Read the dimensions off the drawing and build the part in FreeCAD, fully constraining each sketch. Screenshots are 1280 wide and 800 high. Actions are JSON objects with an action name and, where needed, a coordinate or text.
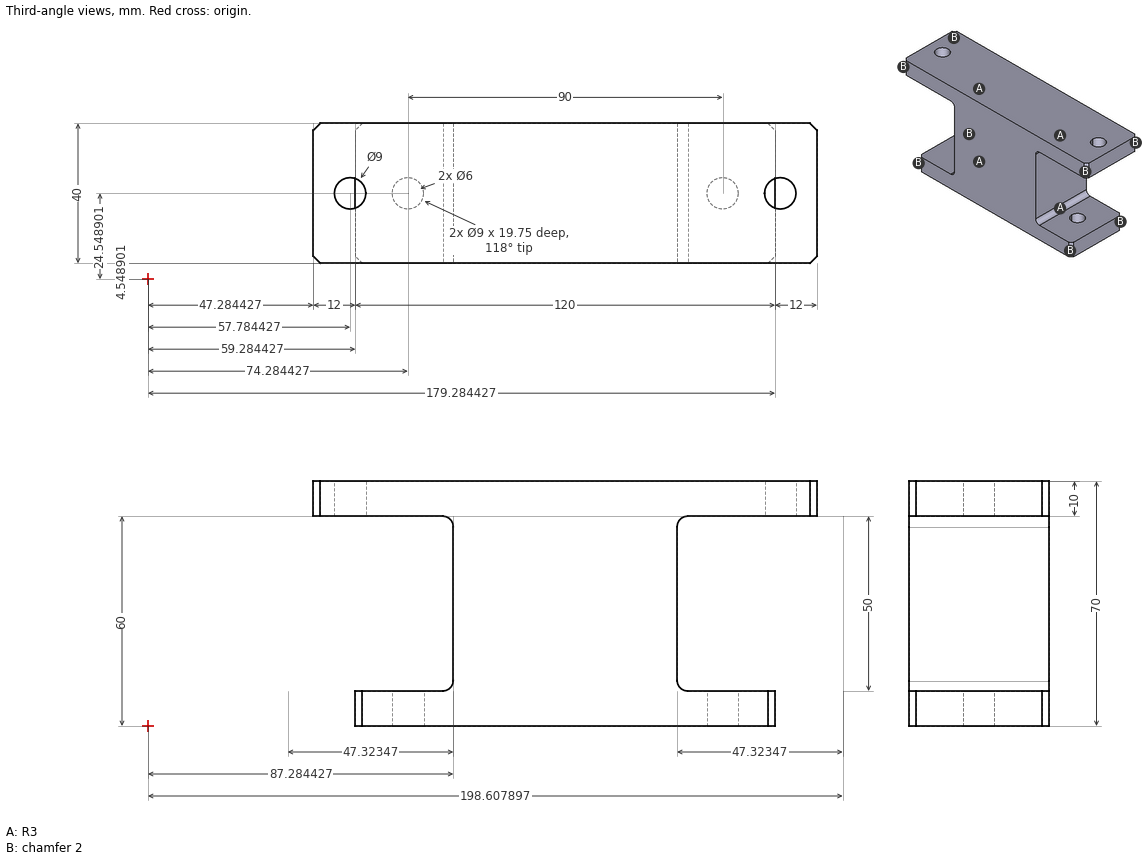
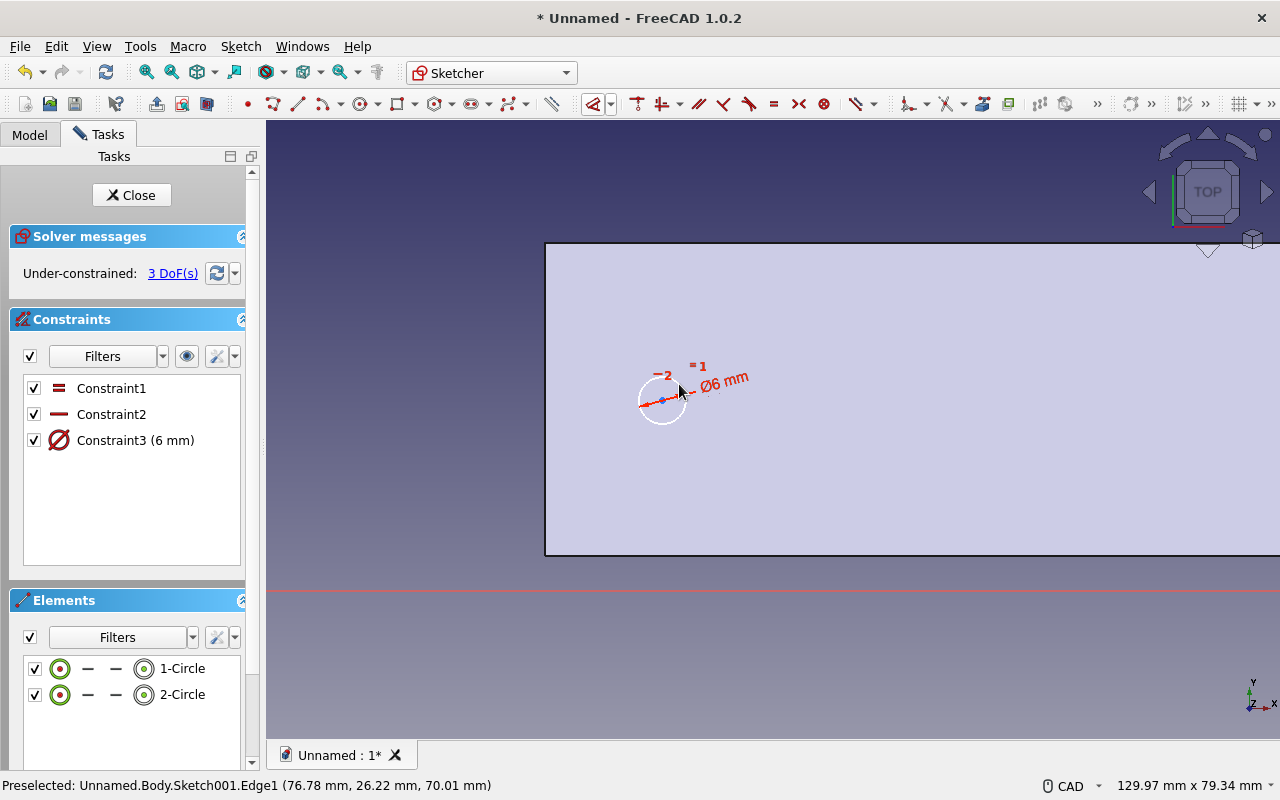
{"action": "left_click", "coordinate": [662, 401]}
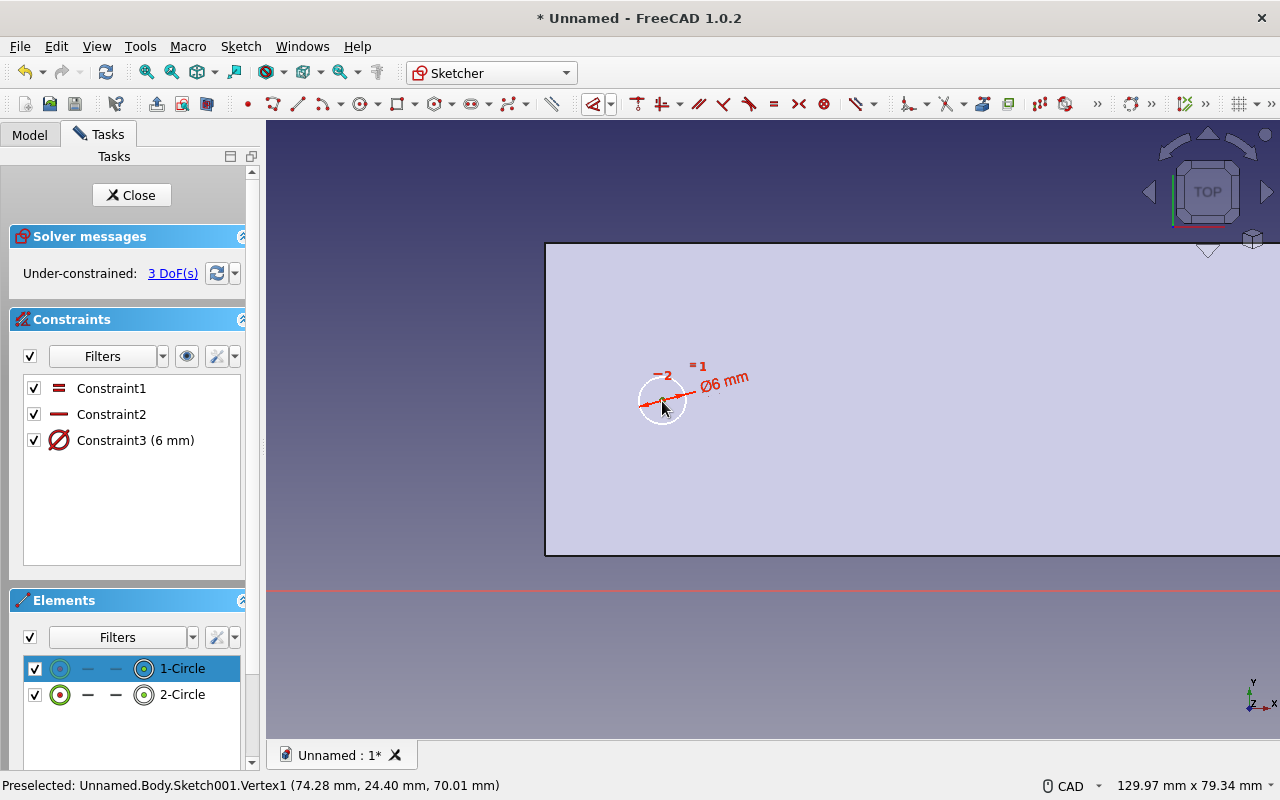
{"action": "scroll", "coordinate": [679, 385], "scroll_direction": "down", "scroll_amount": 4}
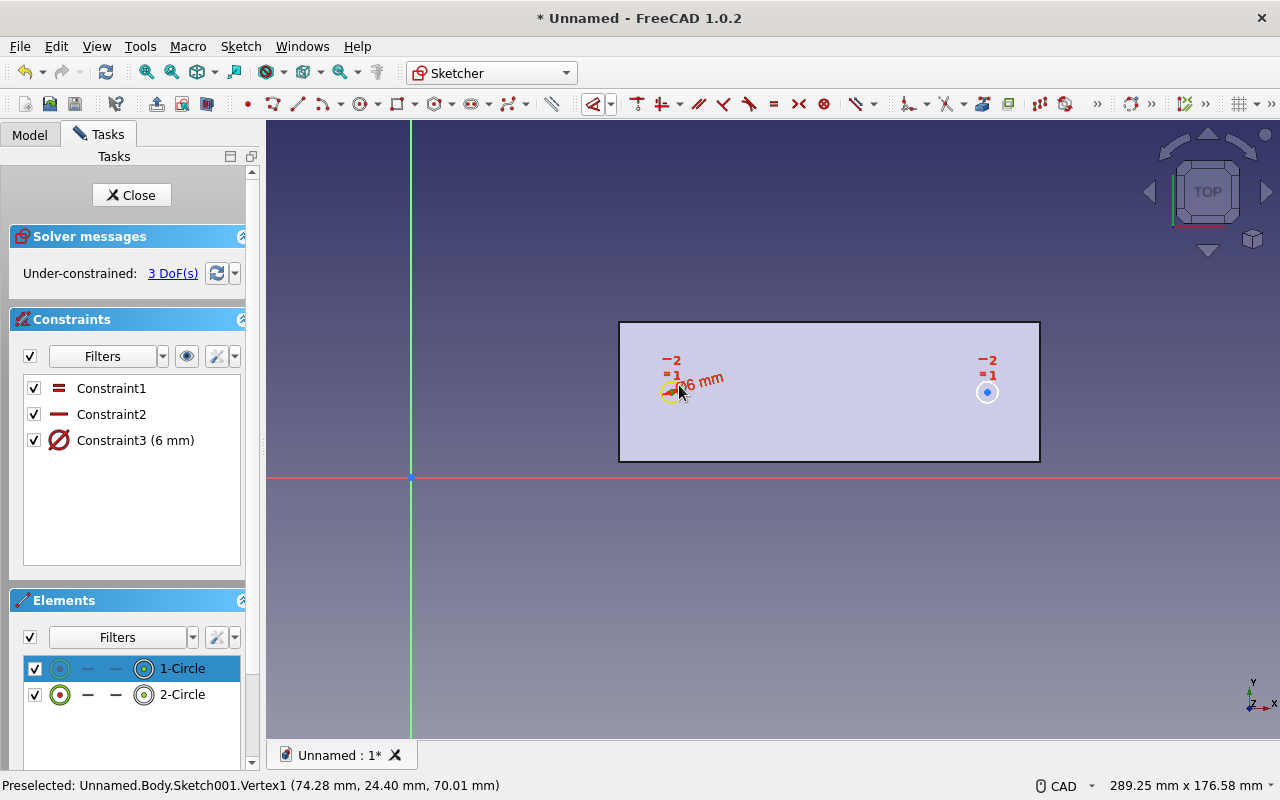
{"action": "left_click", "coordinate": [987, 392]}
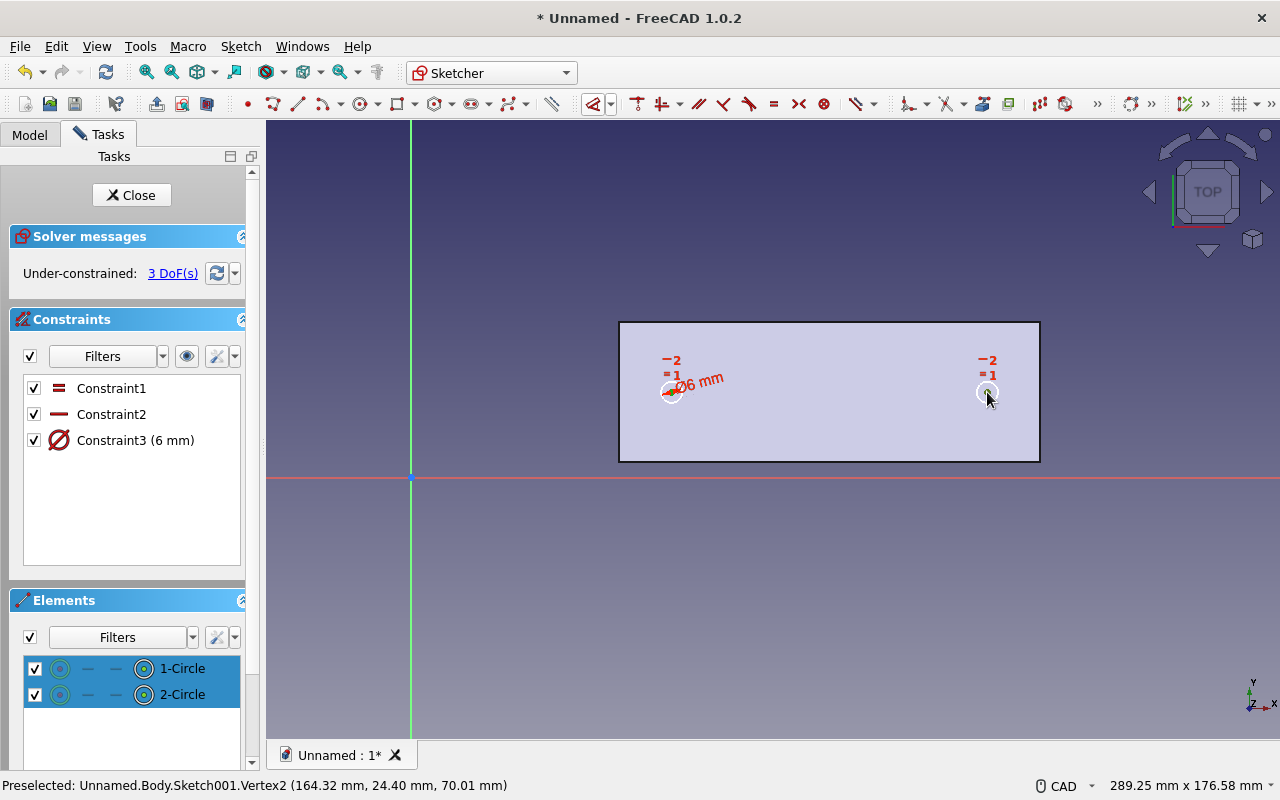
{"action": "key", "text": "l"}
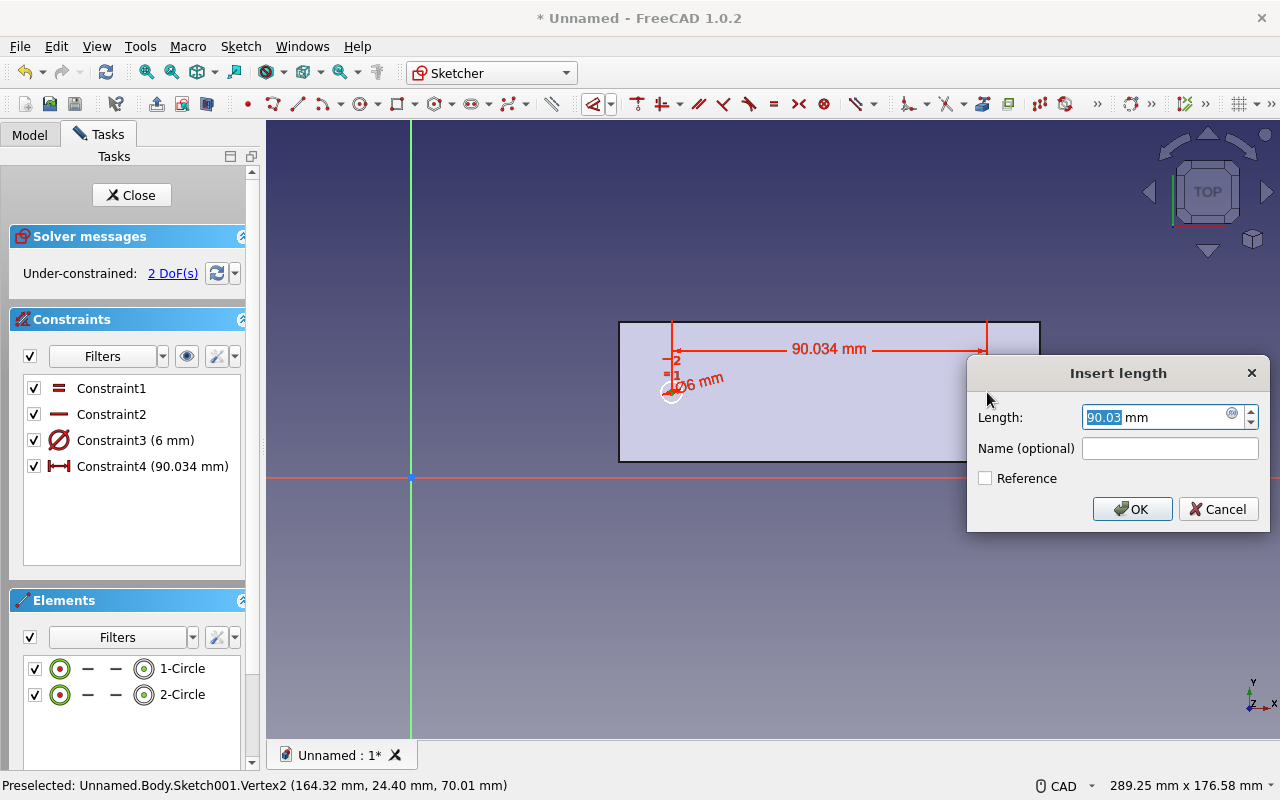
{"action": "type", "text": "90"}
{"action": "key", "text": "Return"}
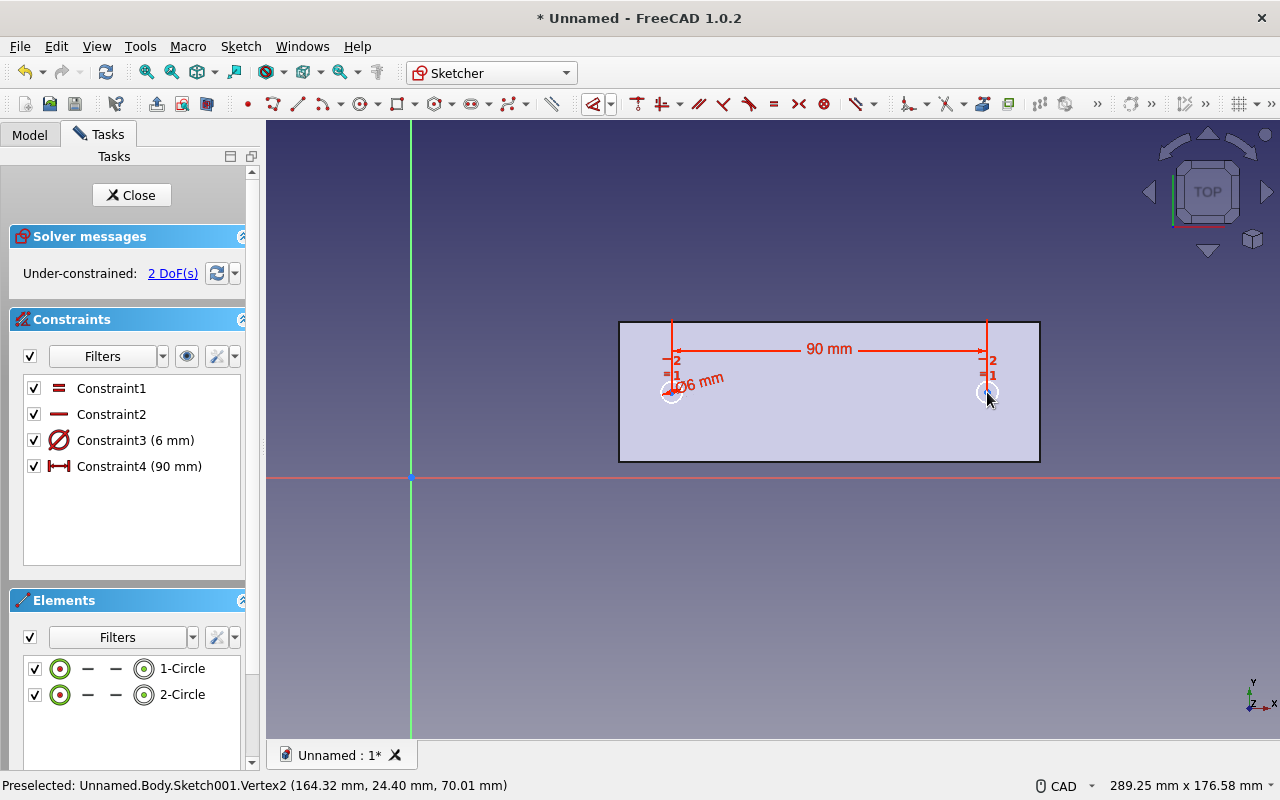
{"action": "left_click", "coordinate": [672, 392]}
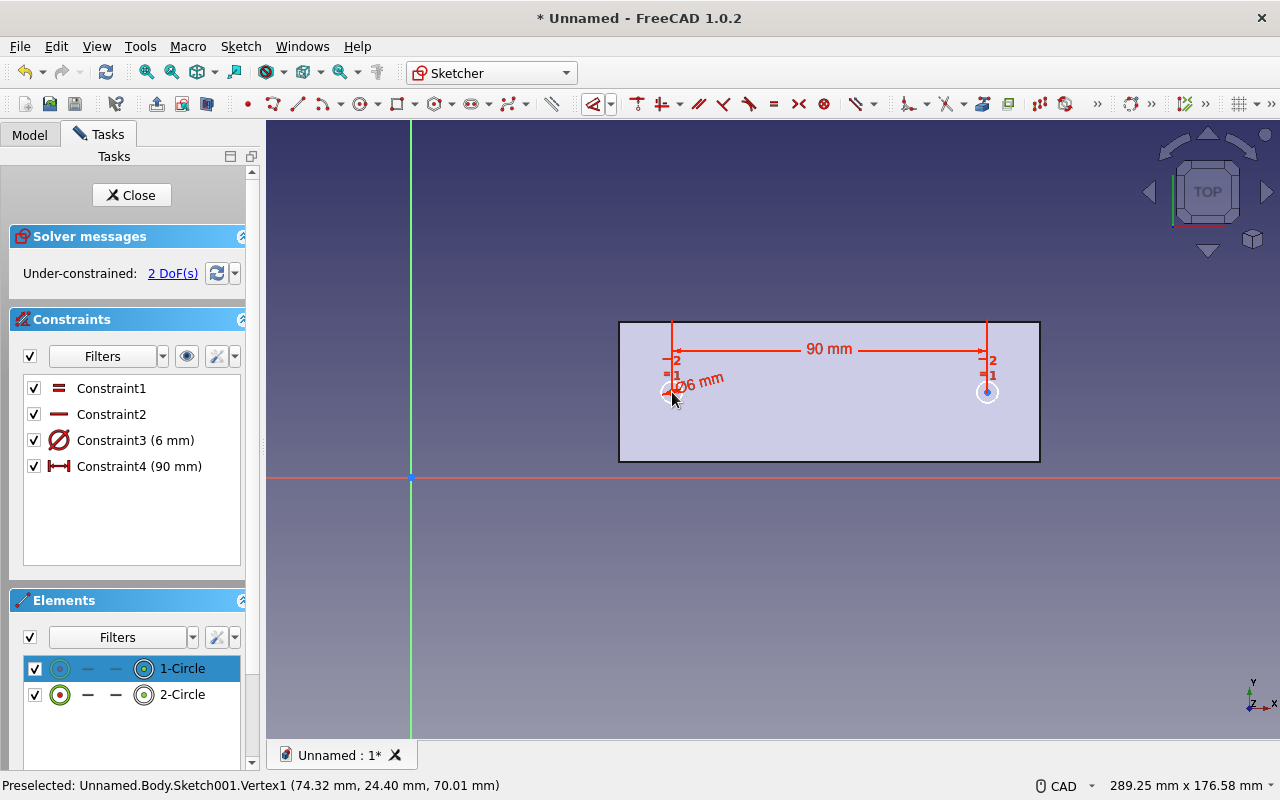
{"action": "key", "text": "l"}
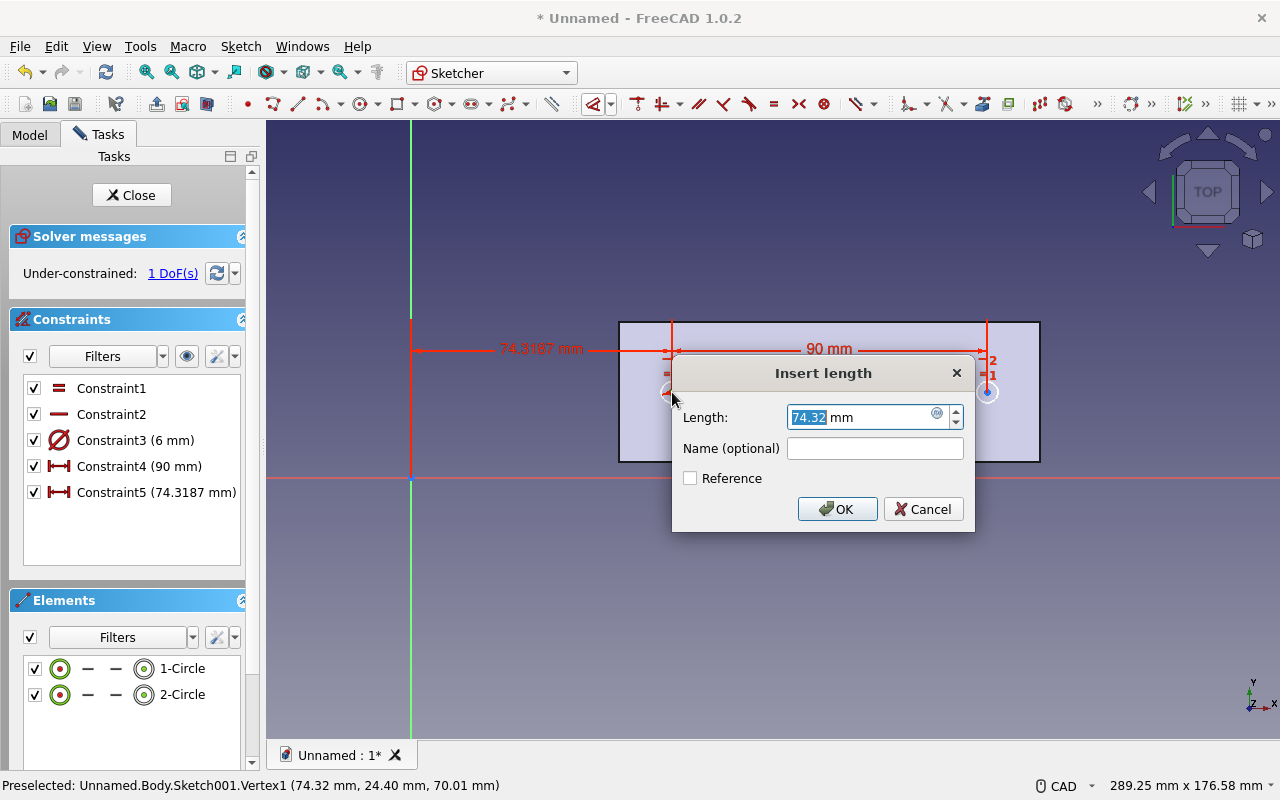
{"action": "type", "text": "74.284427"}
{"action": "key", "text": "Return"}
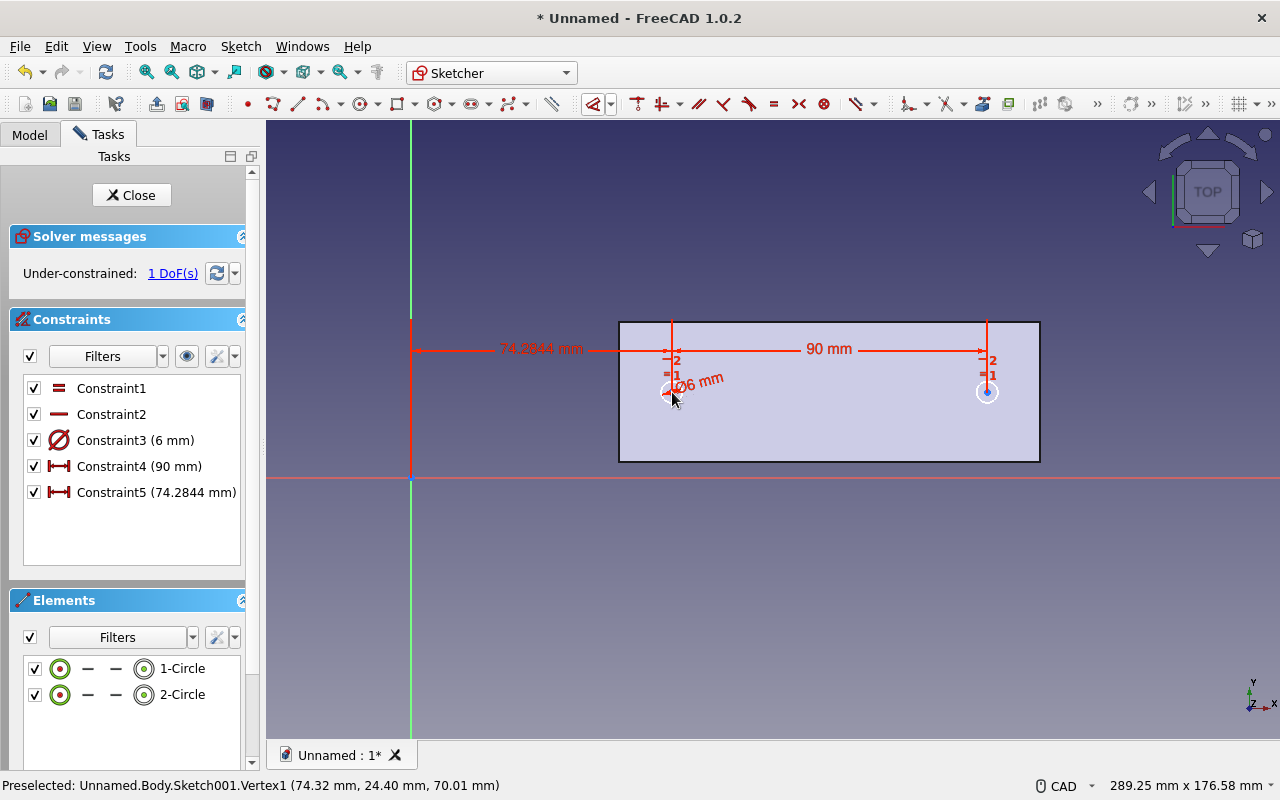
{"action": "left_click", "coordinate": [672, 392]}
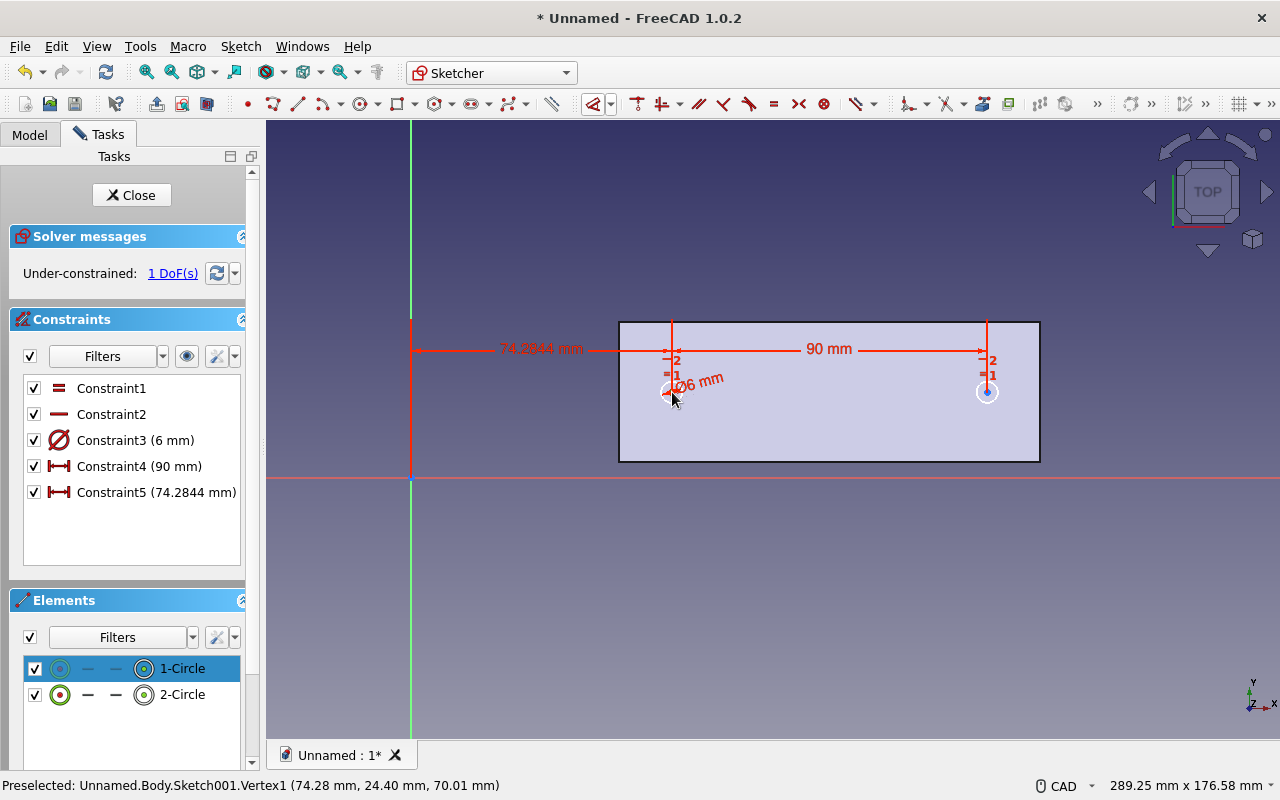
{"action": "left_click", "coordinate": [610, 104]}